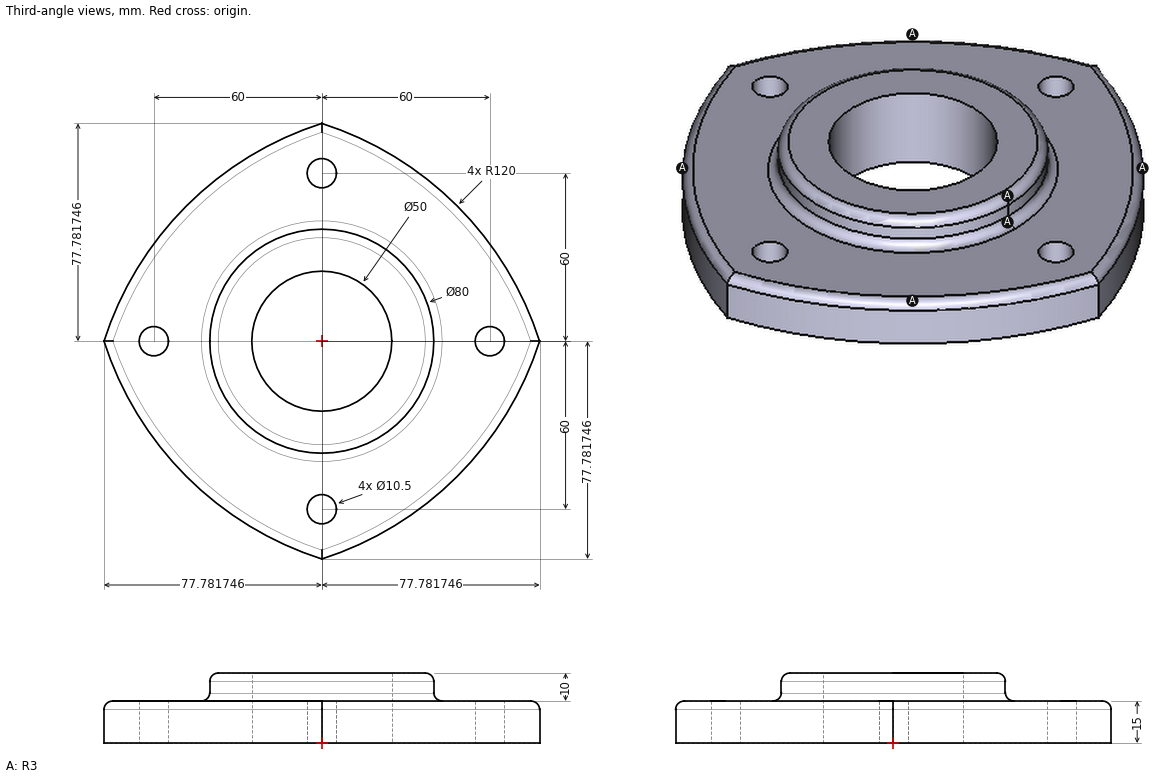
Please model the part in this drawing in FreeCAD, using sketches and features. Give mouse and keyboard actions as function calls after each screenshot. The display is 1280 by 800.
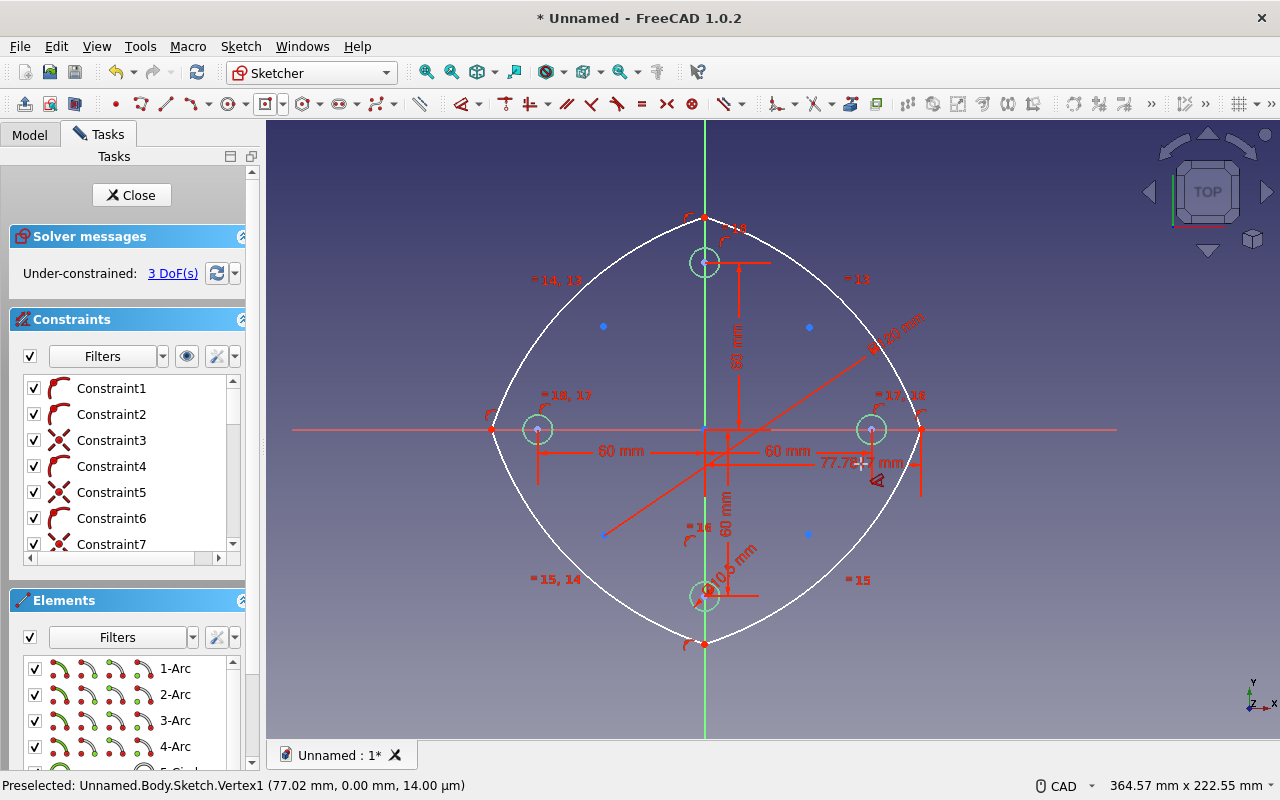
click(705, 217)
click(671, 323)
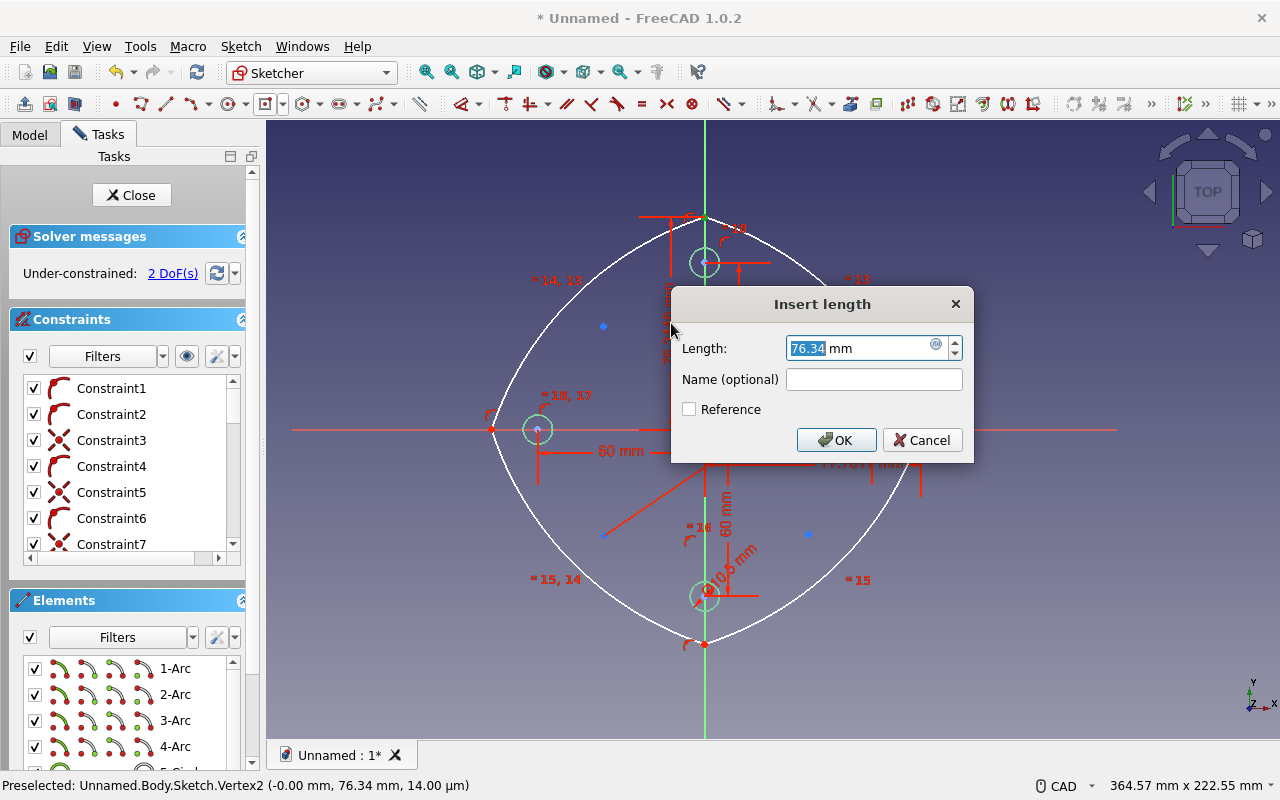
text(77.781746)
key(Return)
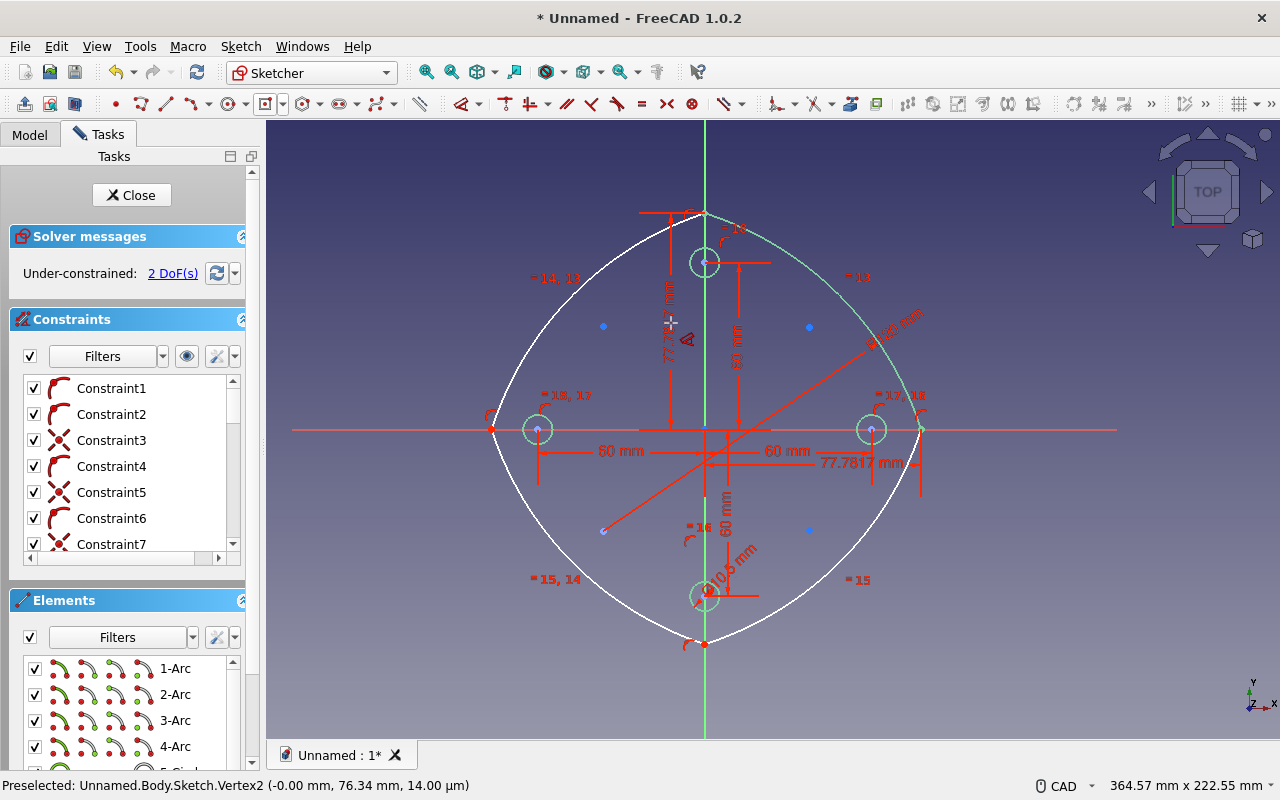
click(492, 430)
click(549, 464)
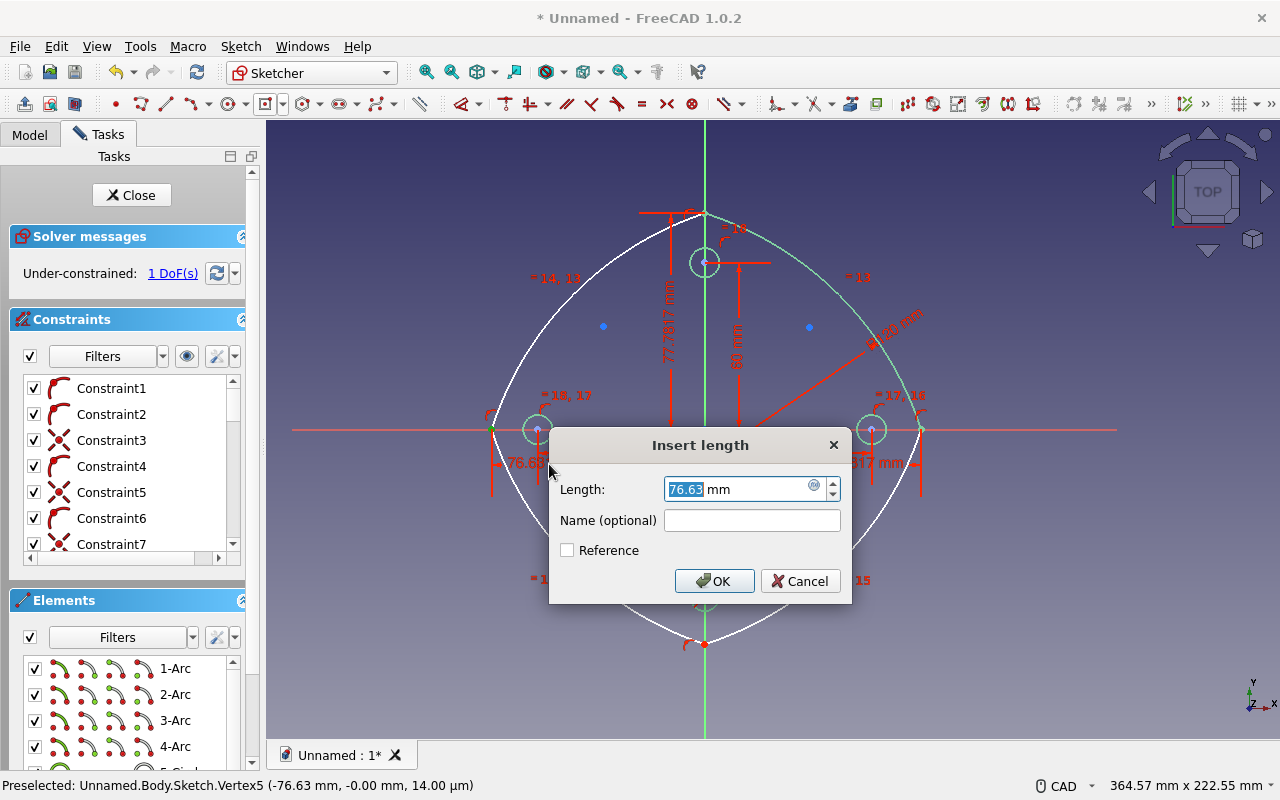
text(77.781746)
key(Return)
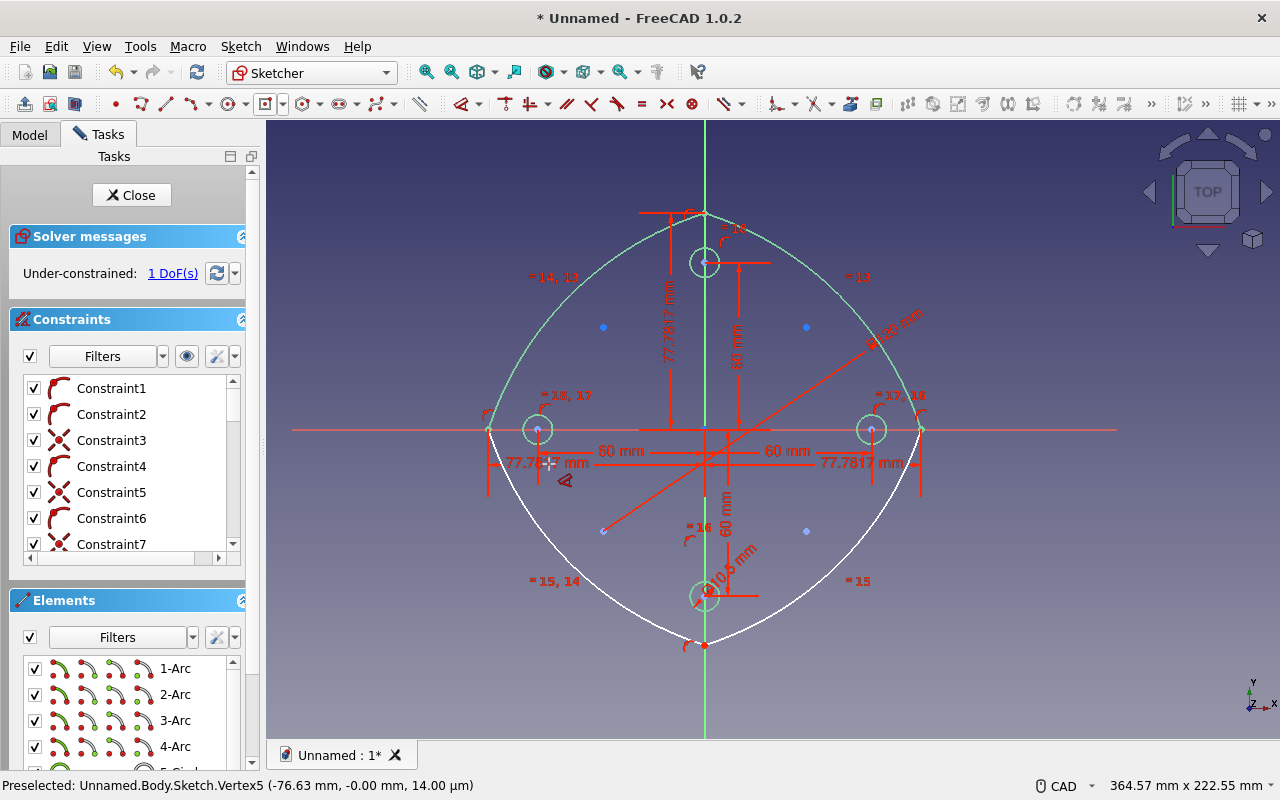
click(705, 645)
click(739, 537)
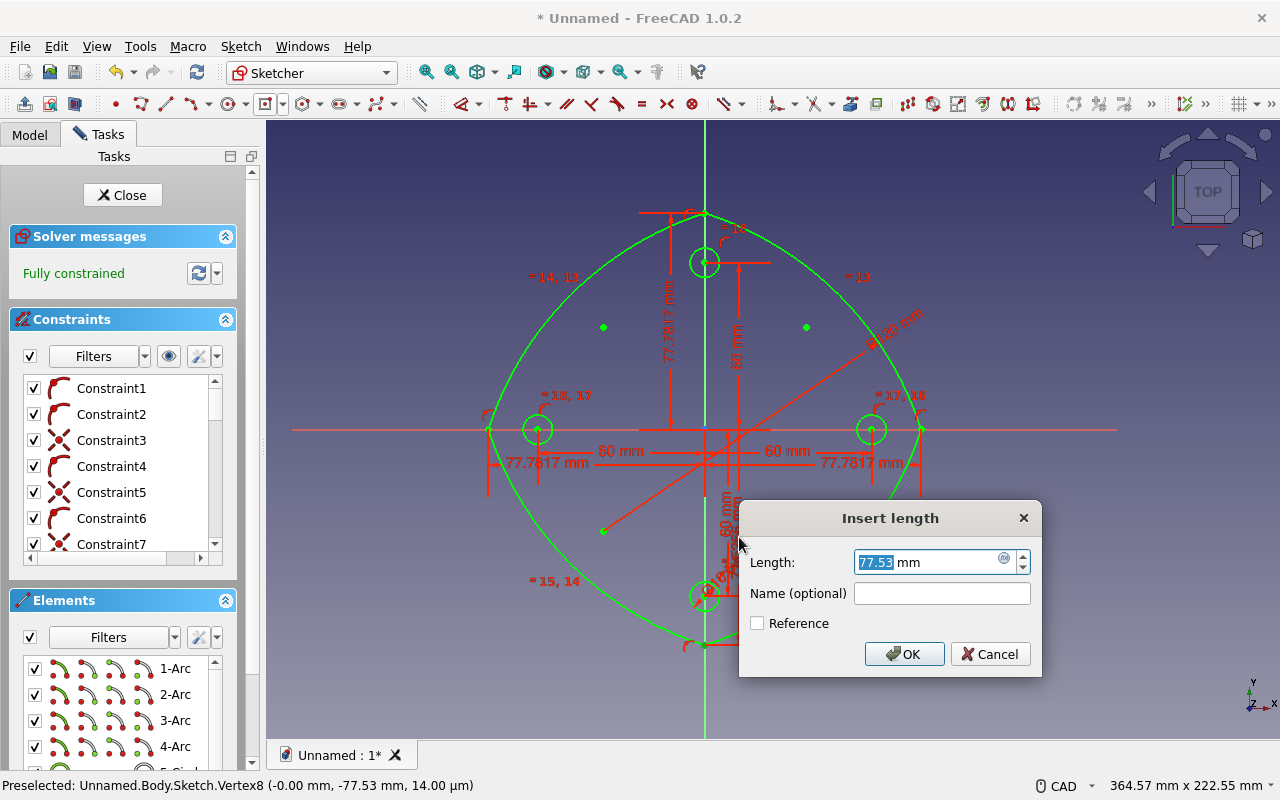
text(77.781746)
key(Return)
key(Escape)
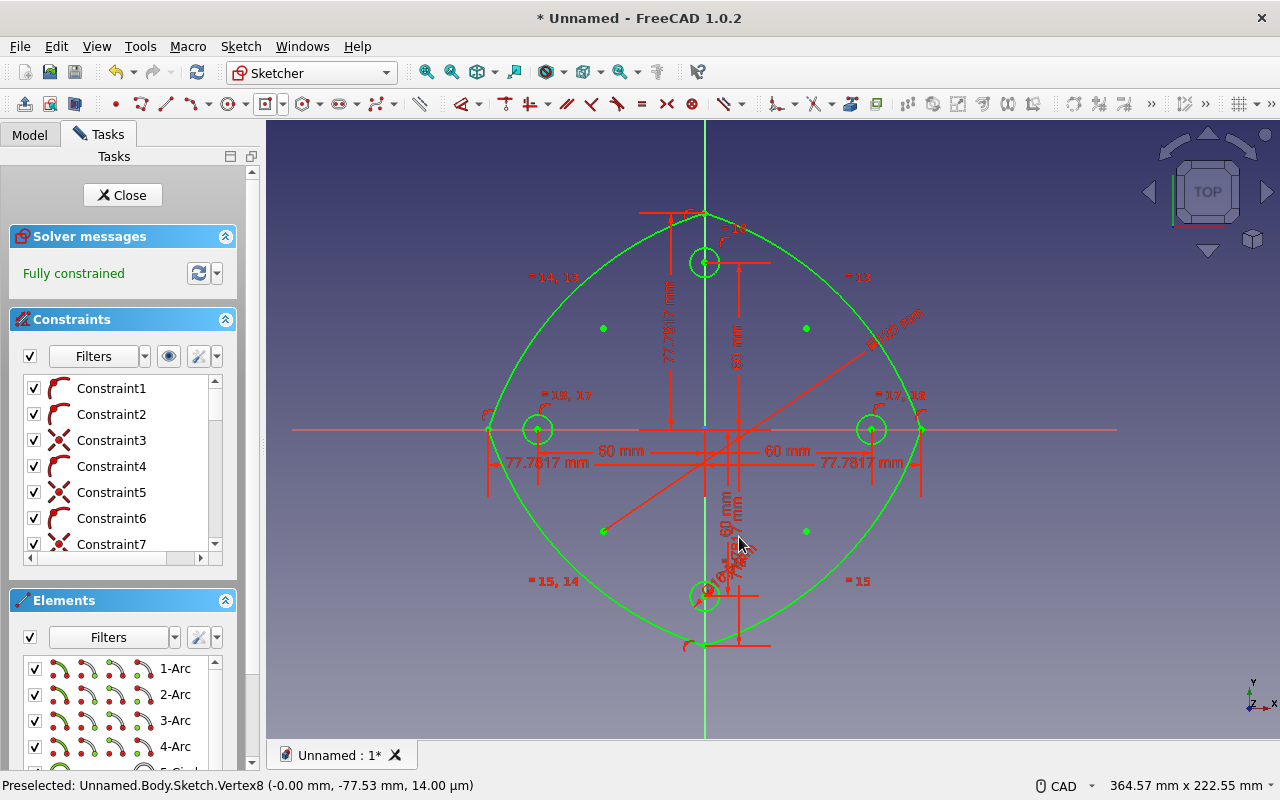
click(123, 195)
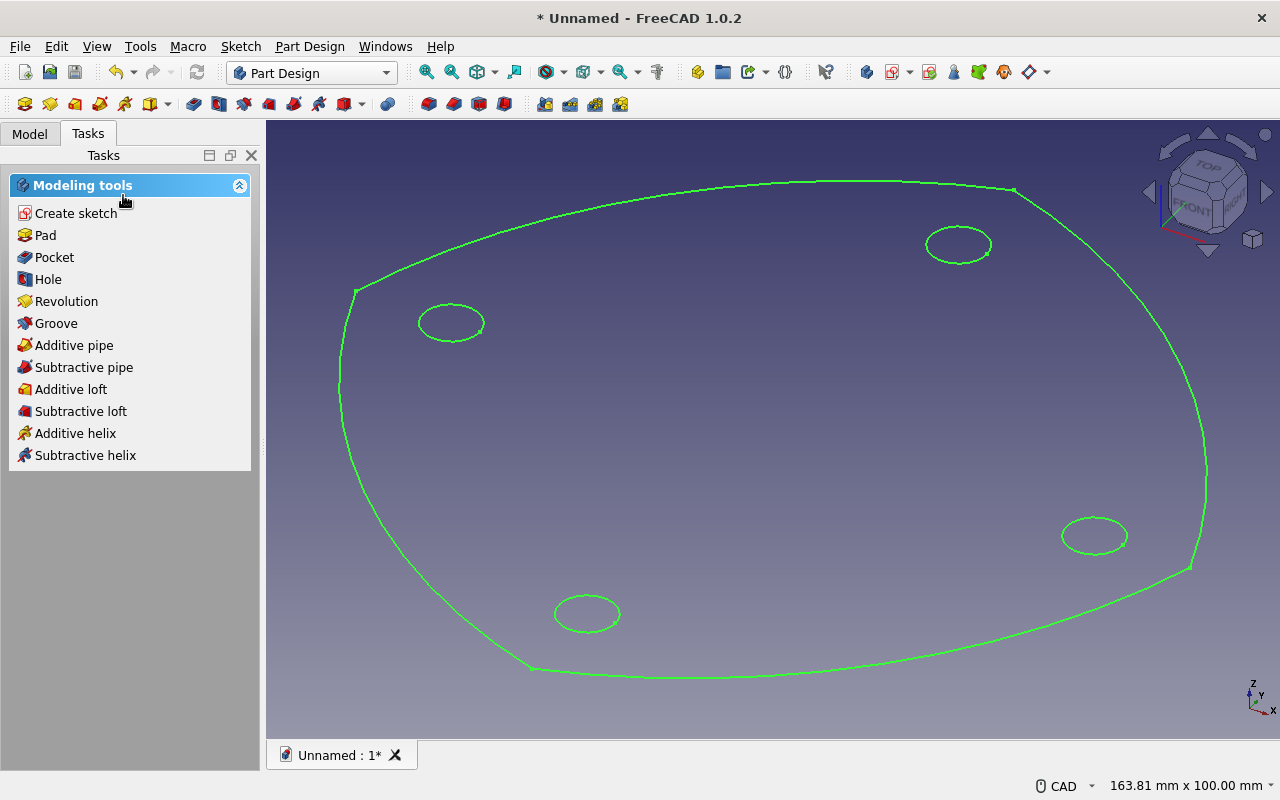
click(25, 104)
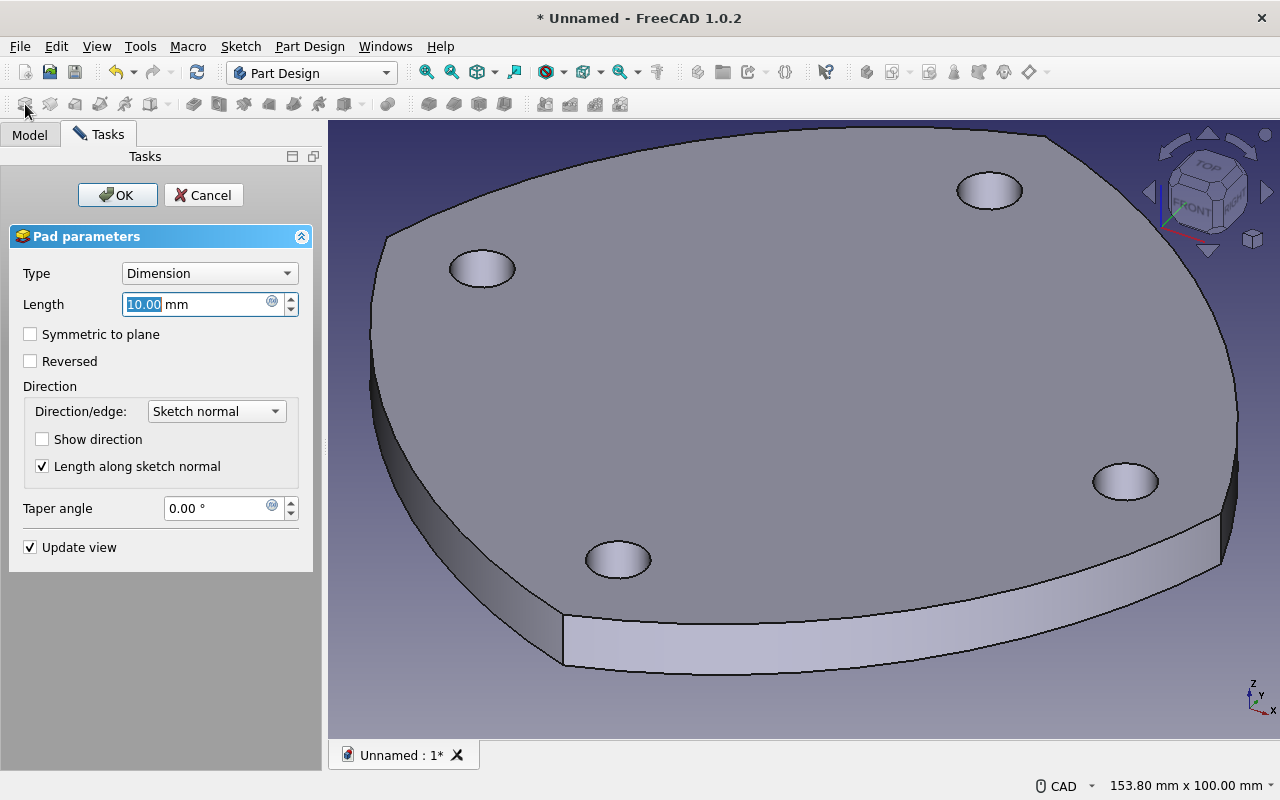
text(15)
key(Tab)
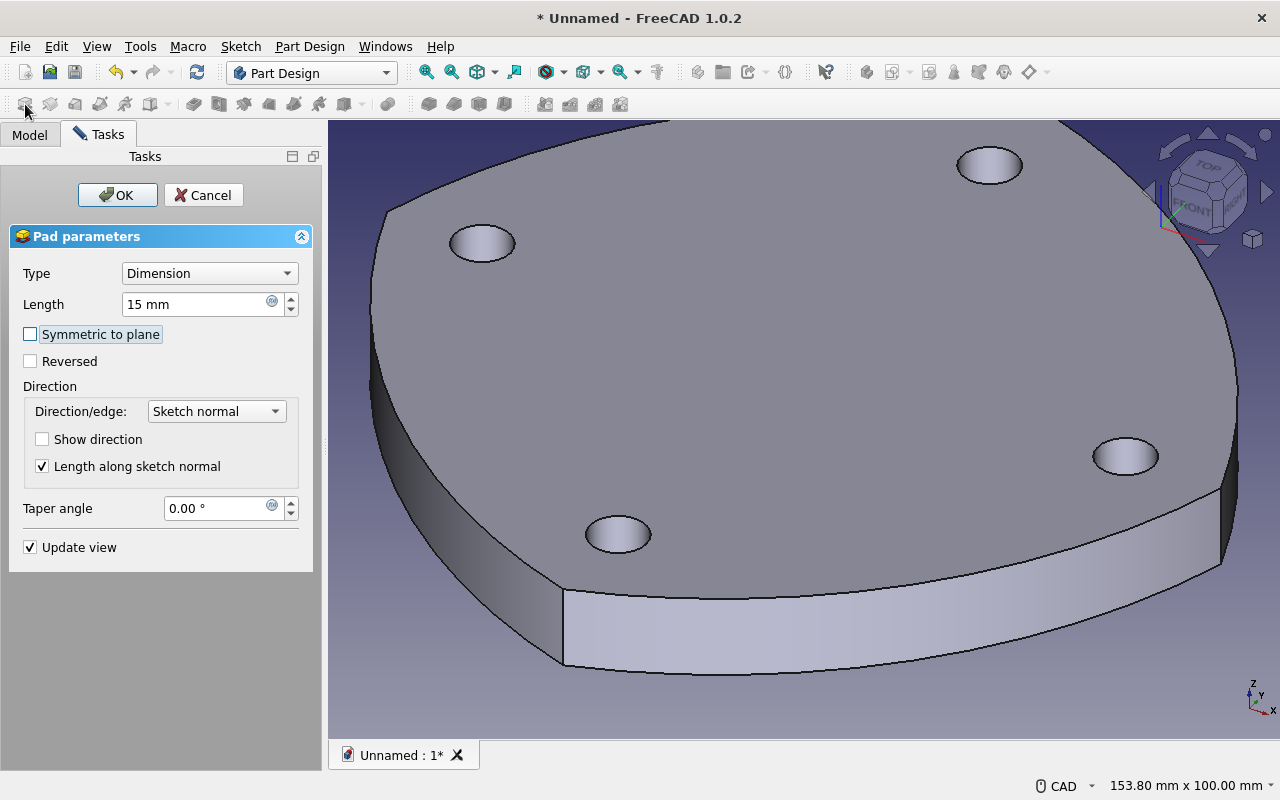
click(118, 195)